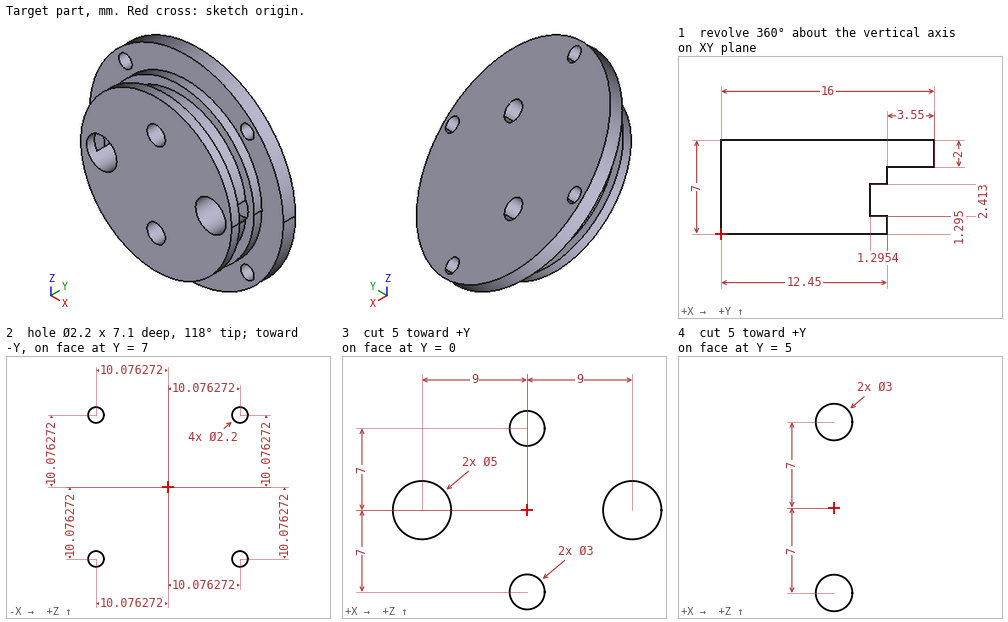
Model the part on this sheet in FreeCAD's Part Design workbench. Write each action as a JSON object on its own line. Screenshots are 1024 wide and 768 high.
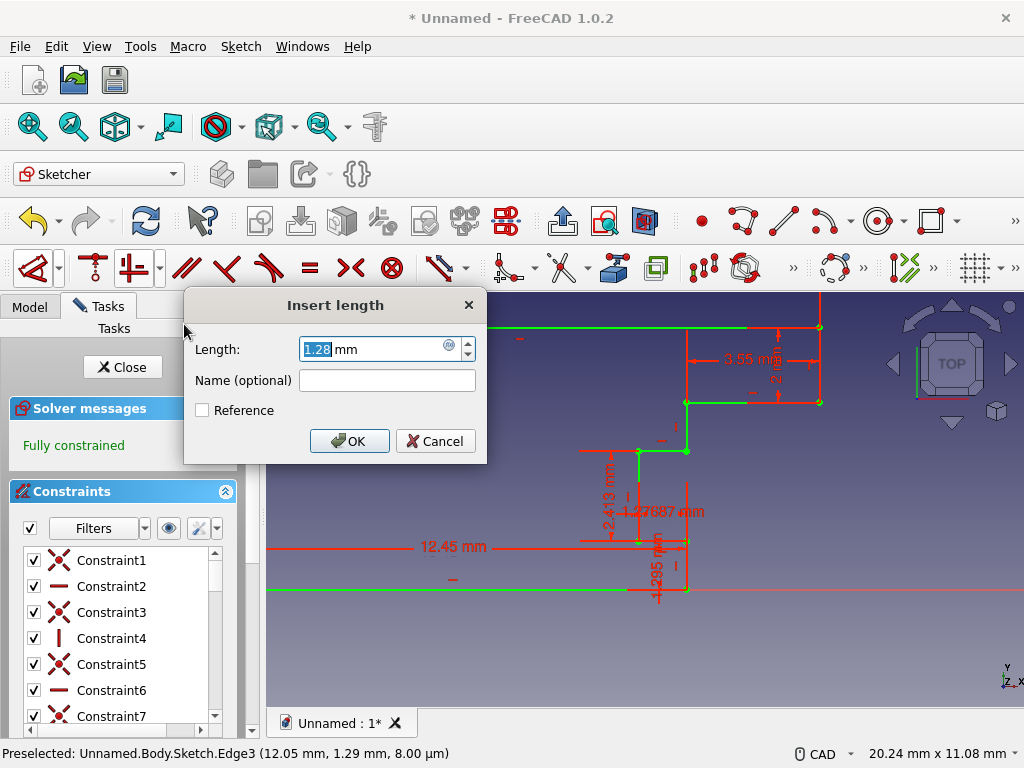
{"action": "type", "text": "1.2954"}
{"action": "key", "text": "Return"}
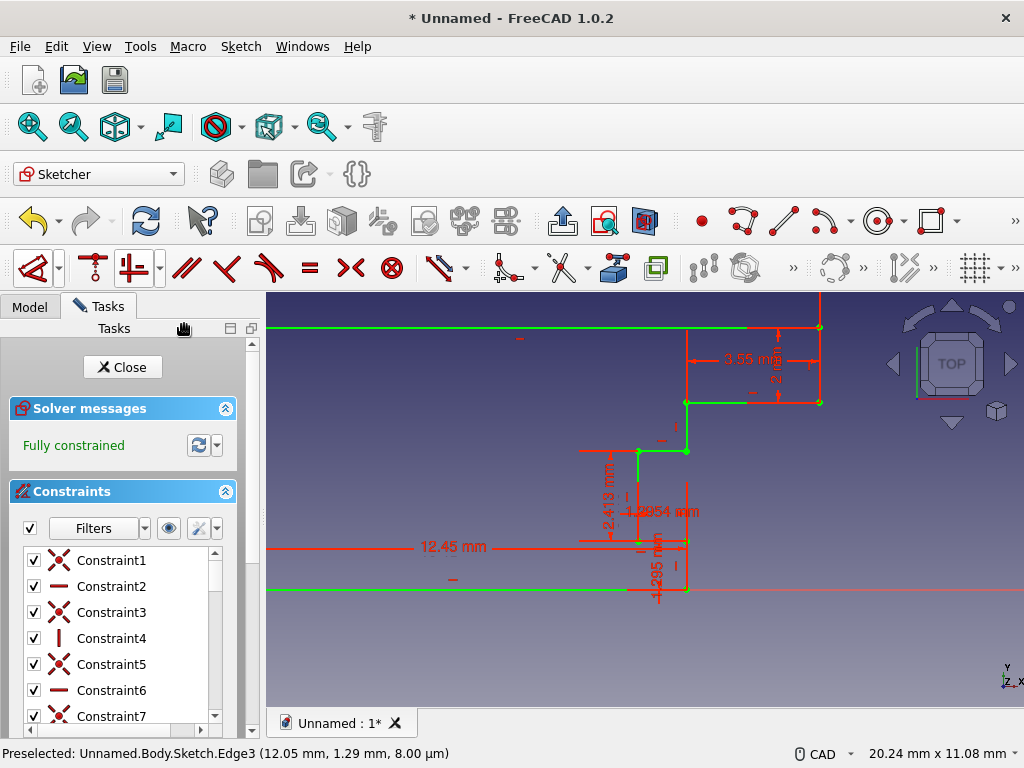
{"action": "left_click", "coordinate": [123, 367]}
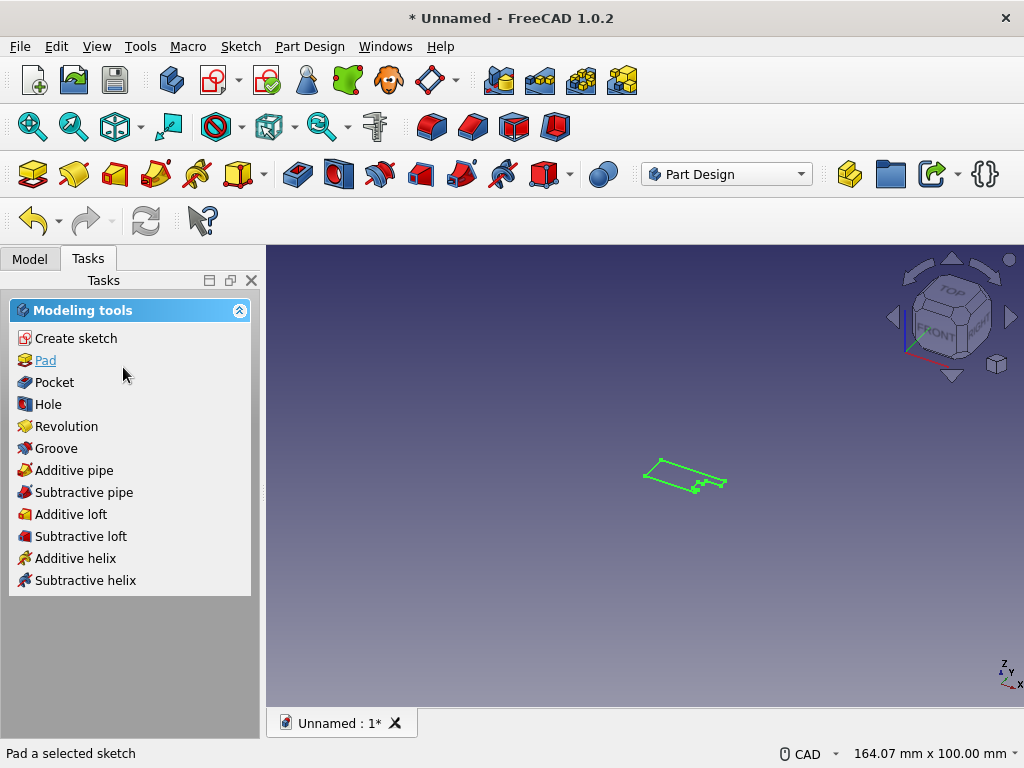
{"action": "left_click", "coordinate": [74, 174]}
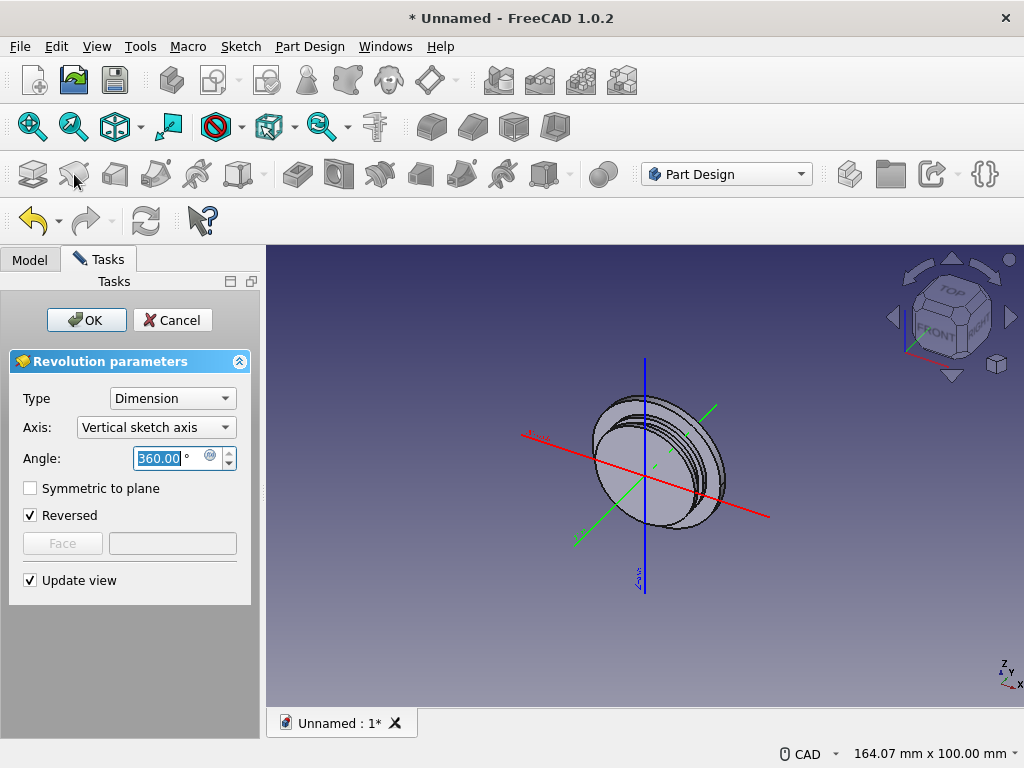
{"action": "left_click", "coordinate": [87, 320]}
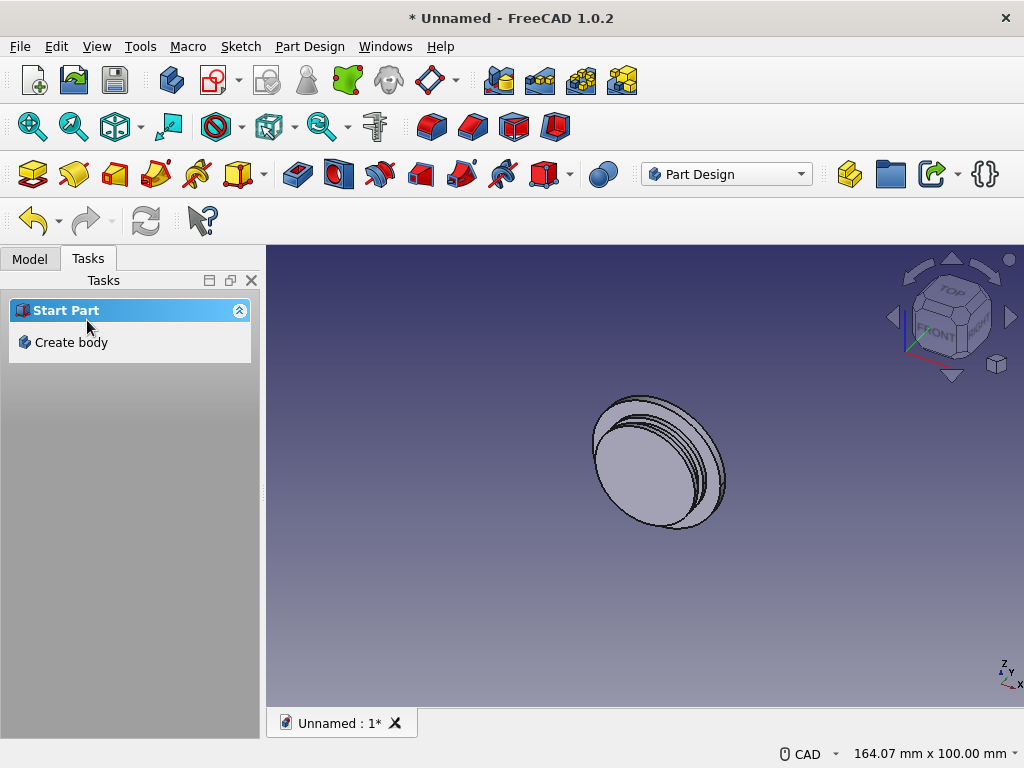
{"action": "left_click", "coordinate": [33, 128]}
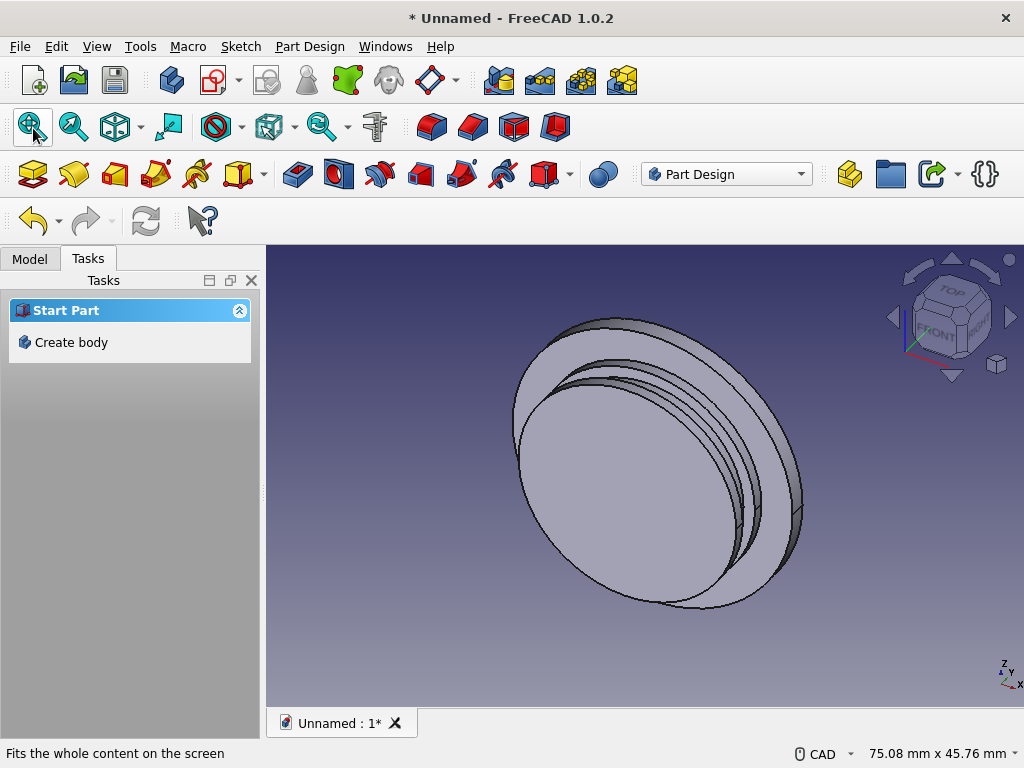
{"action": "key", "text": "4"}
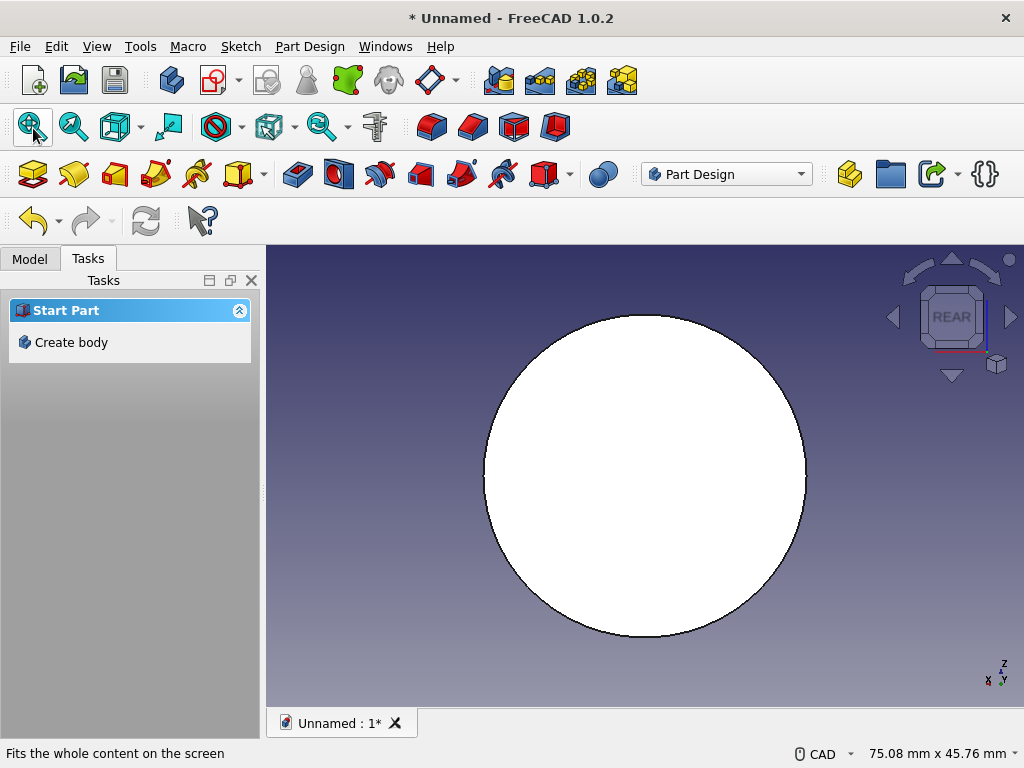
{"action": "left_click", "coordinate": [645, 475]}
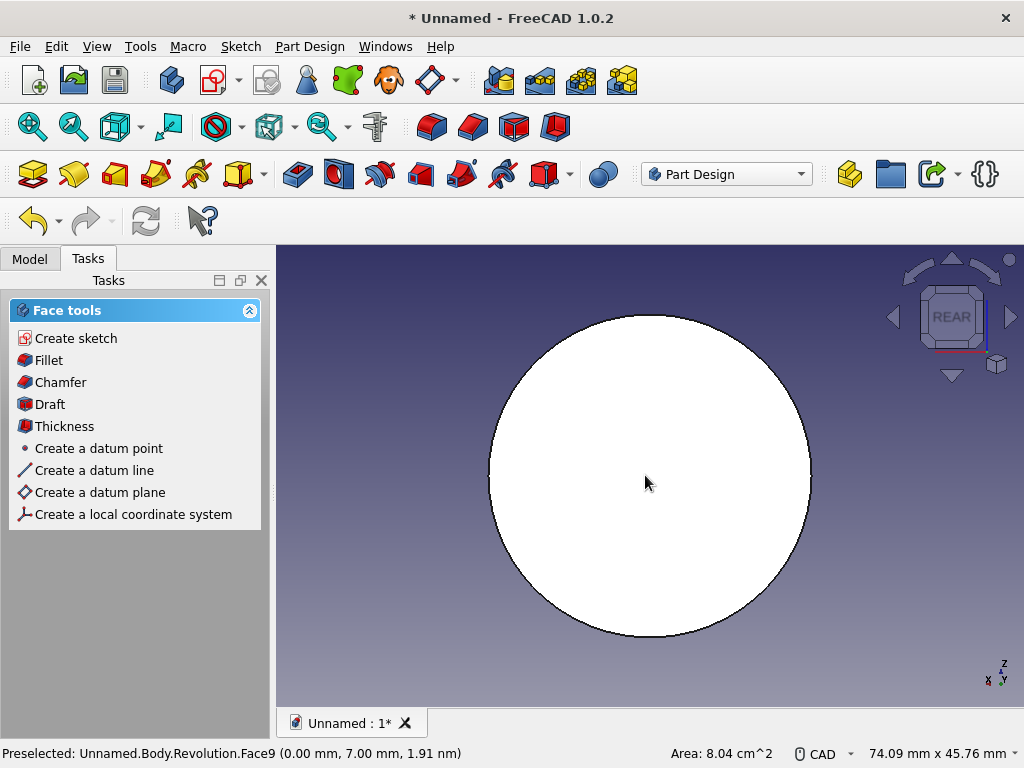
{"action": "left_click", "coordinate": [212, 80]}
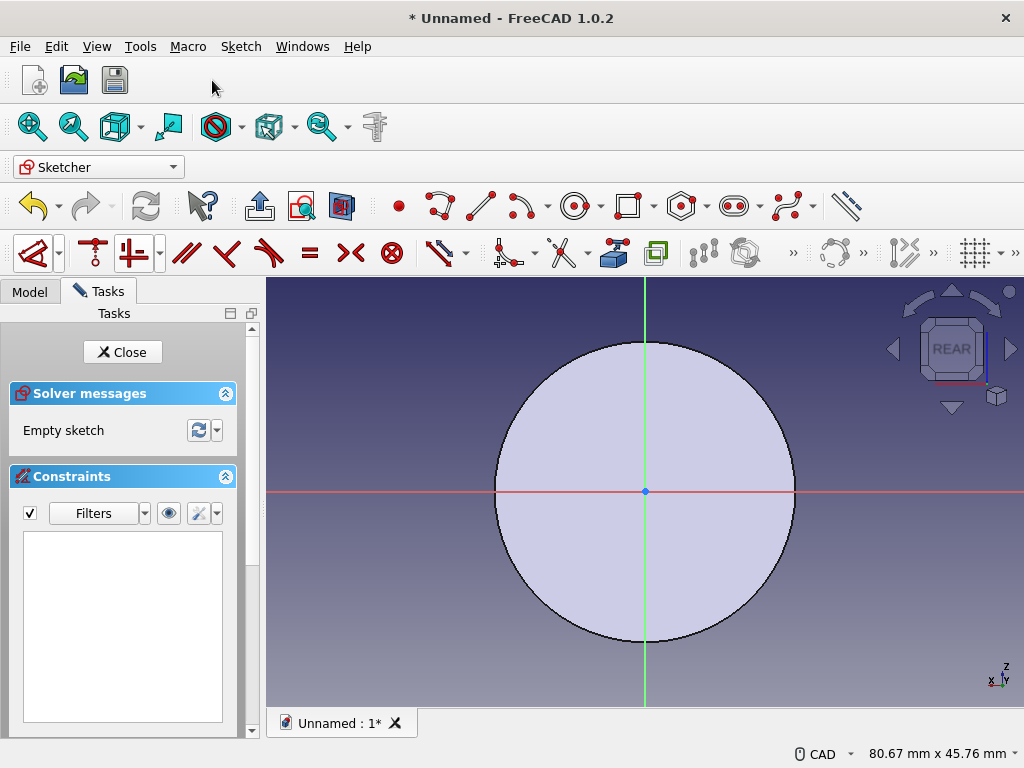
{"action": "left_click", "coordinate": [574, 206]}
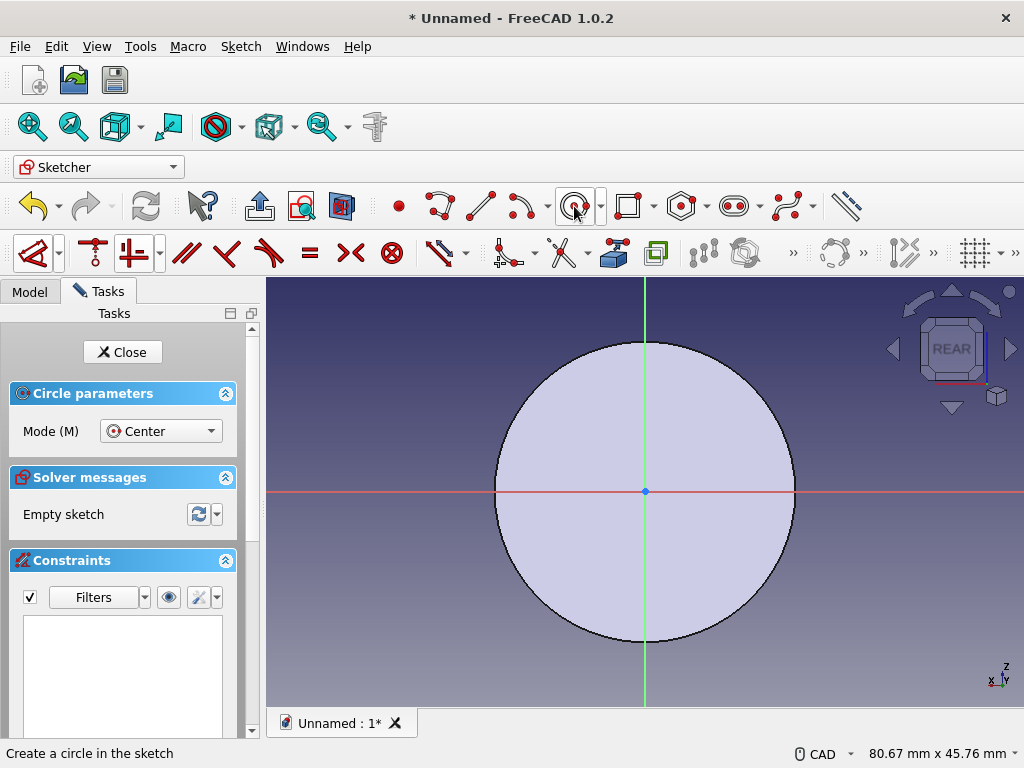
{"action": "scroll", "coordinate": [740, 397], "scroll_direction": "up", "scroll_amount": 4}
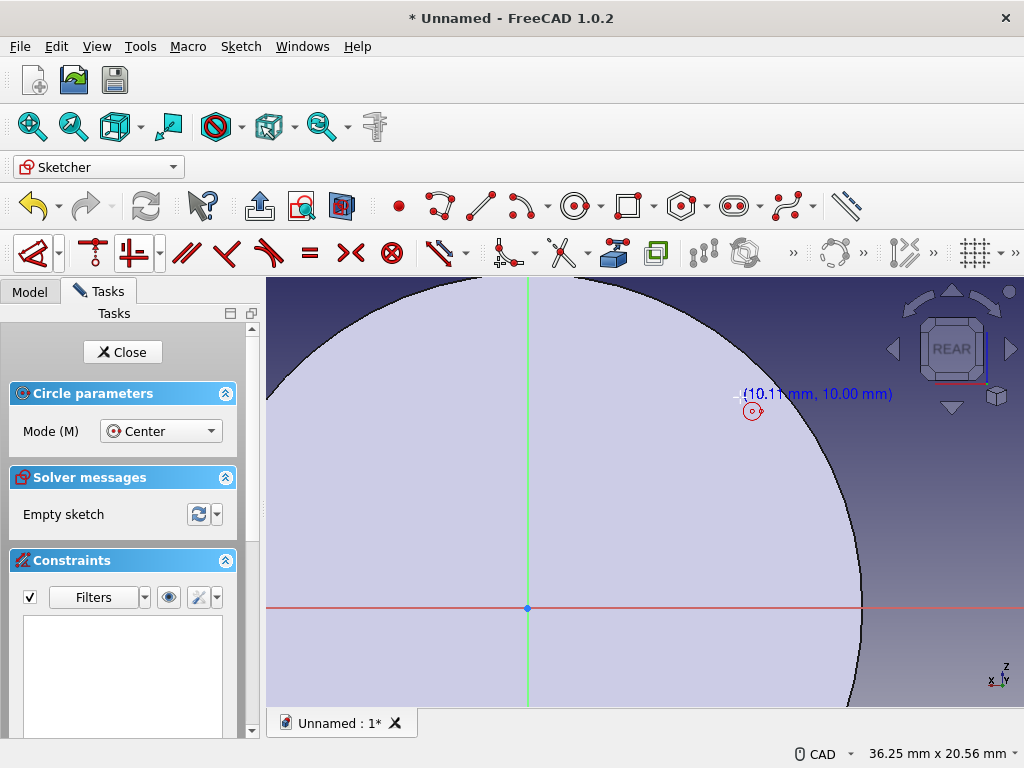
{"action": "left_click", "coordinate": [739, 397]}
{"action": "mouse_move", "coordinate": [755, 381]}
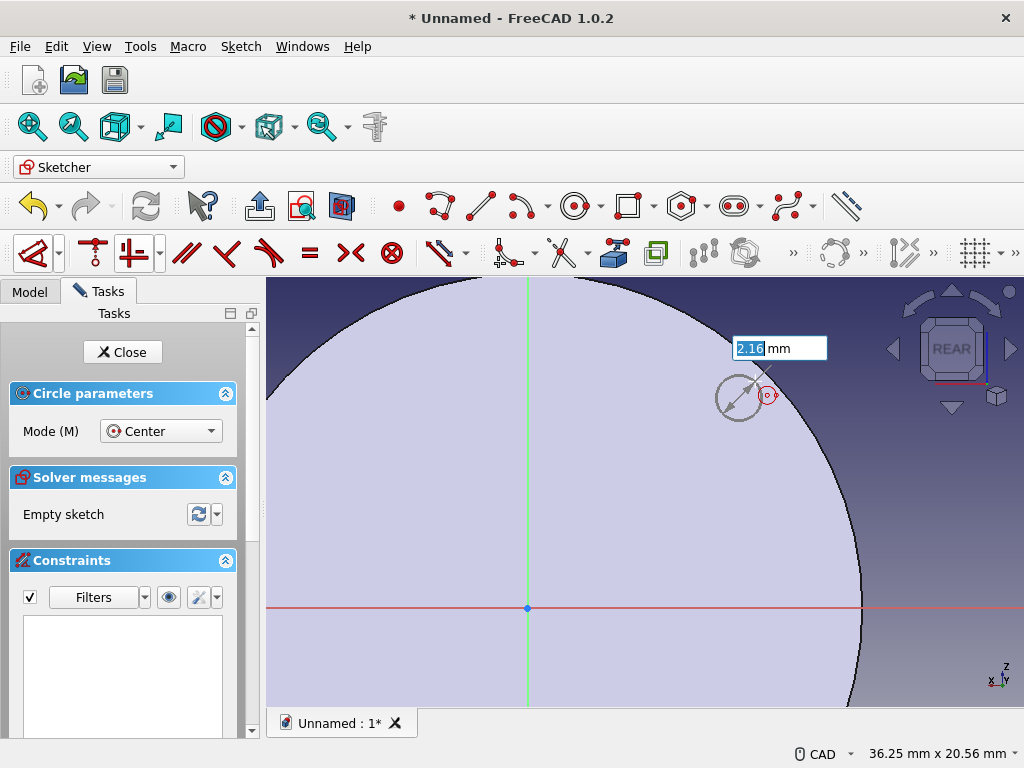
{"action": "type", "text": "2.2"}
{"action": "key", "text": "Return"}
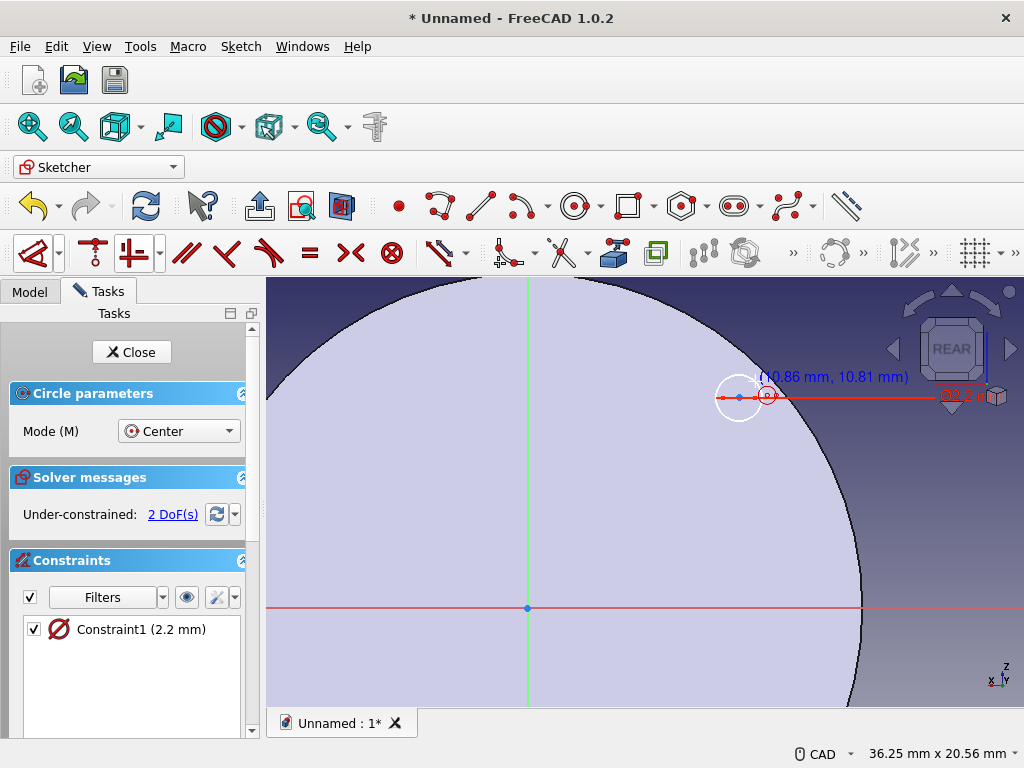
{"action": "scroll", "coordinate": [636, 351], "scroll_direction": "down", "scroll_amount": 3}